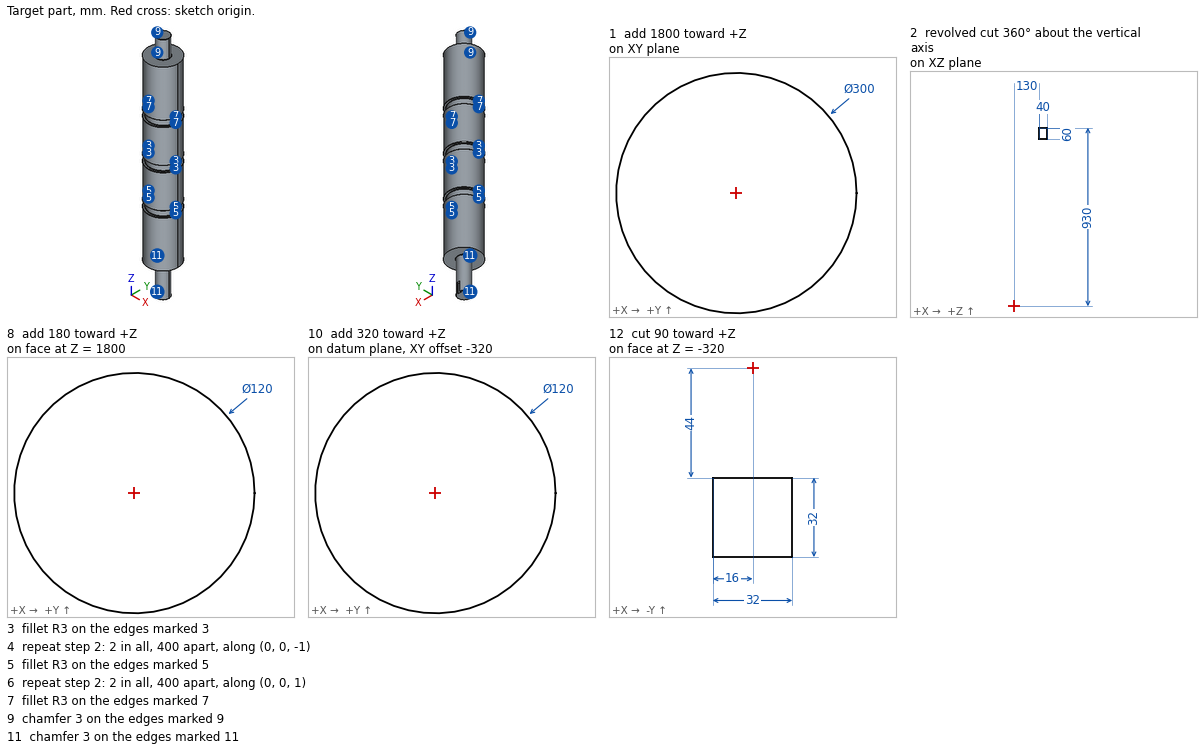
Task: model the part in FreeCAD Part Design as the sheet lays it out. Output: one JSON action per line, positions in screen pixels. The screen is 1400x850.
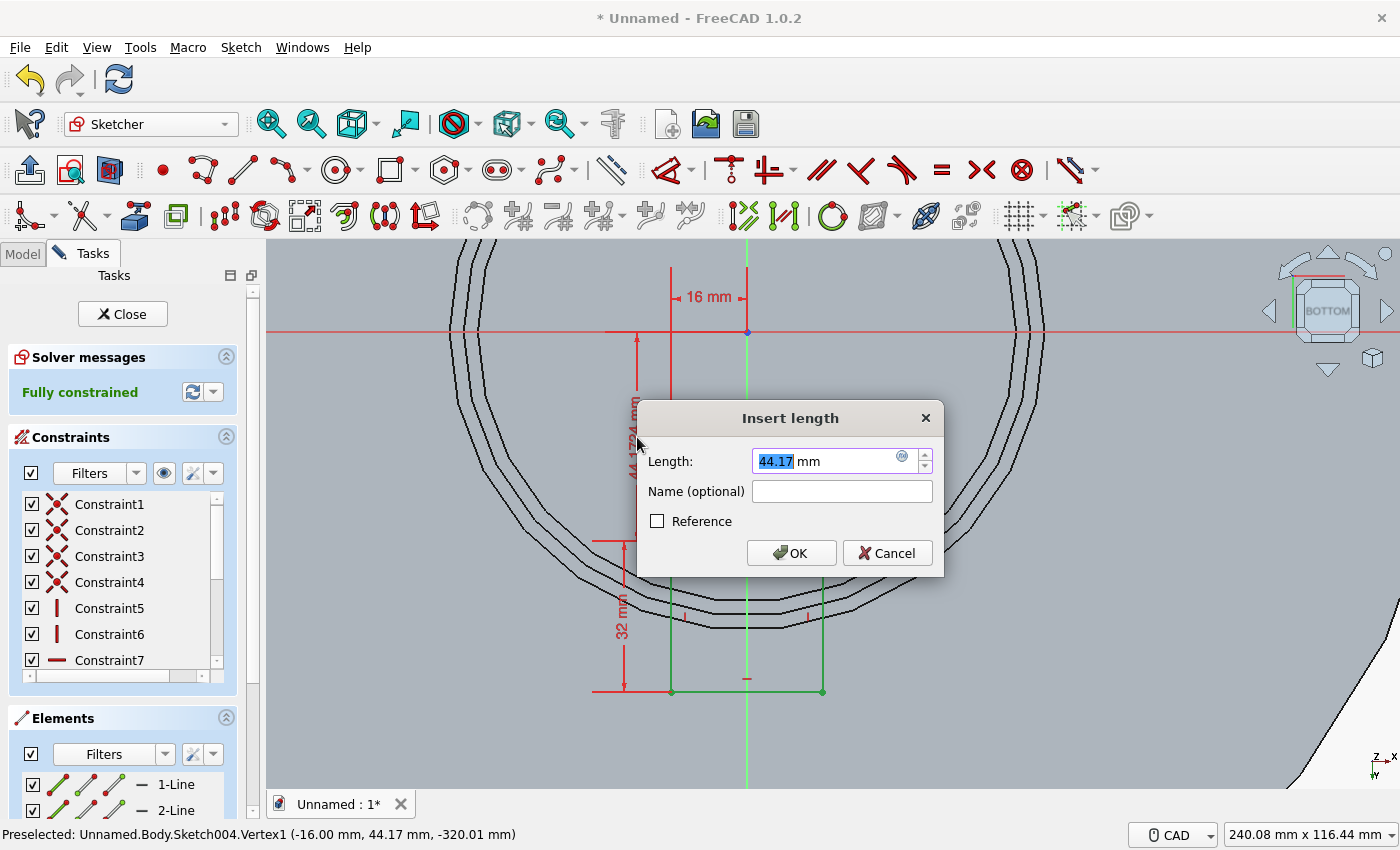
{"action": "type", "text": "44"}
{"action": "key", "text": "Return"}
{"action": "key", "text": "Escape"}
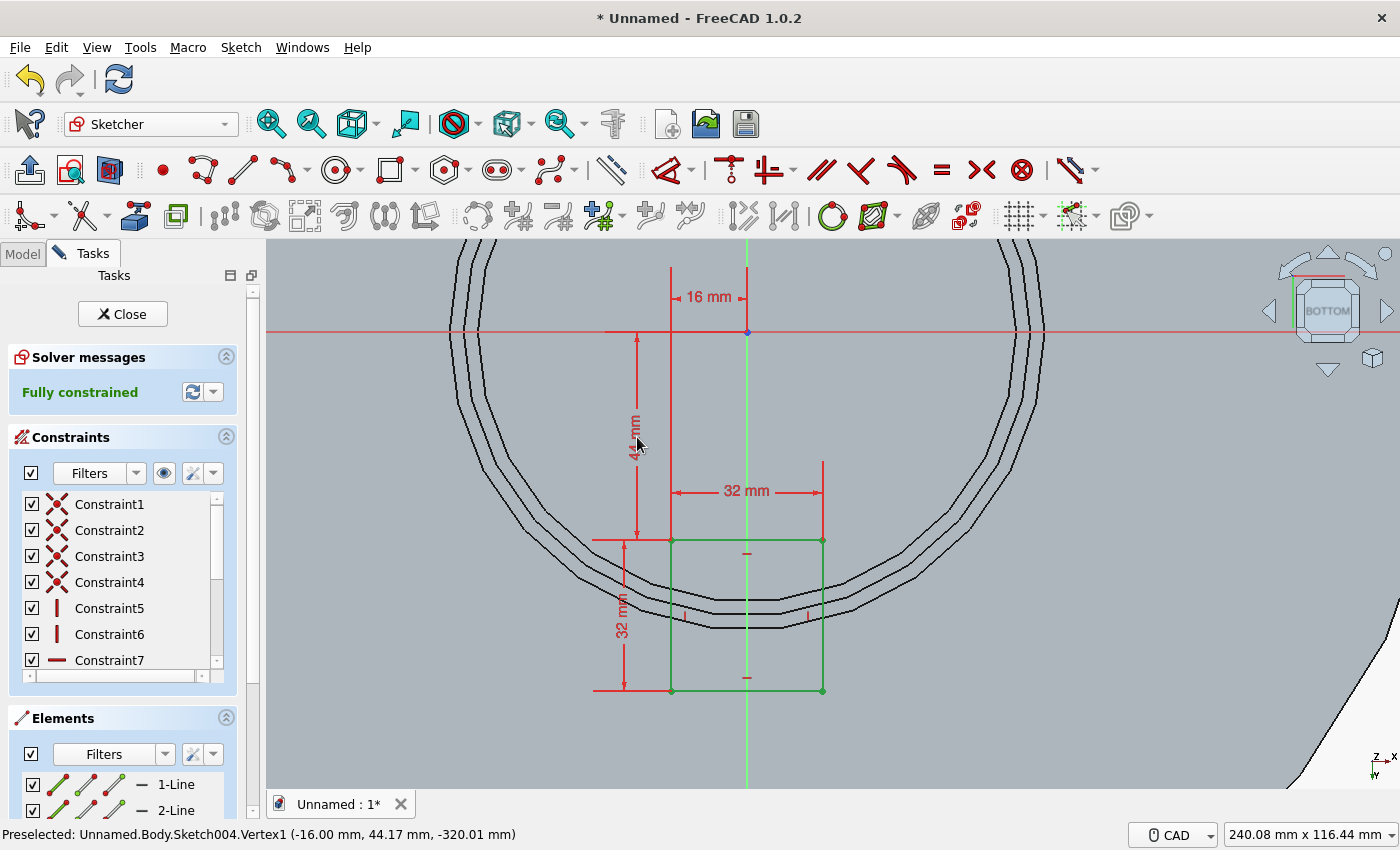
{"action": "left_click", "coordinate": [123, 314]}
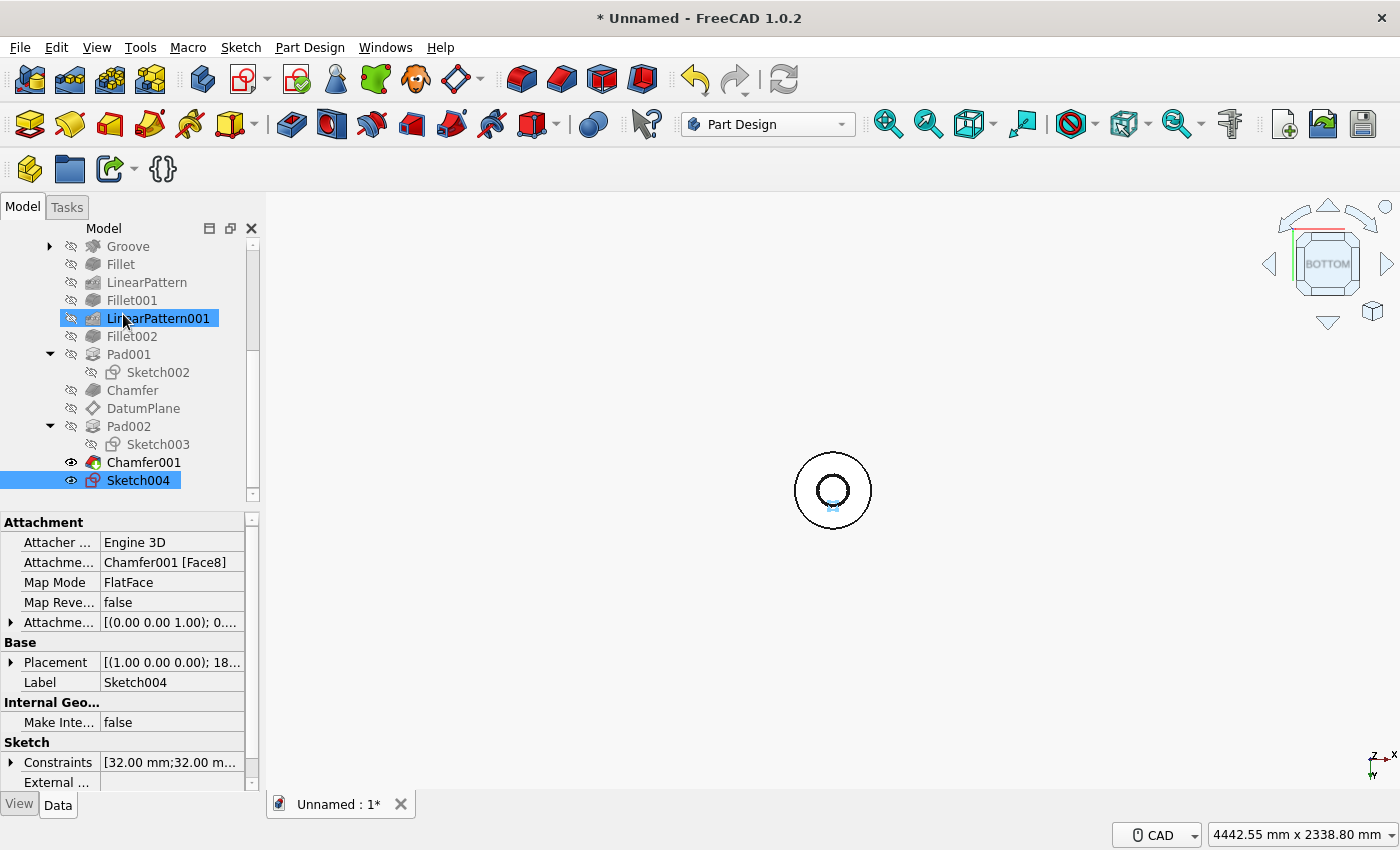
{"action": "left_click", "coordinate": [292, 124]}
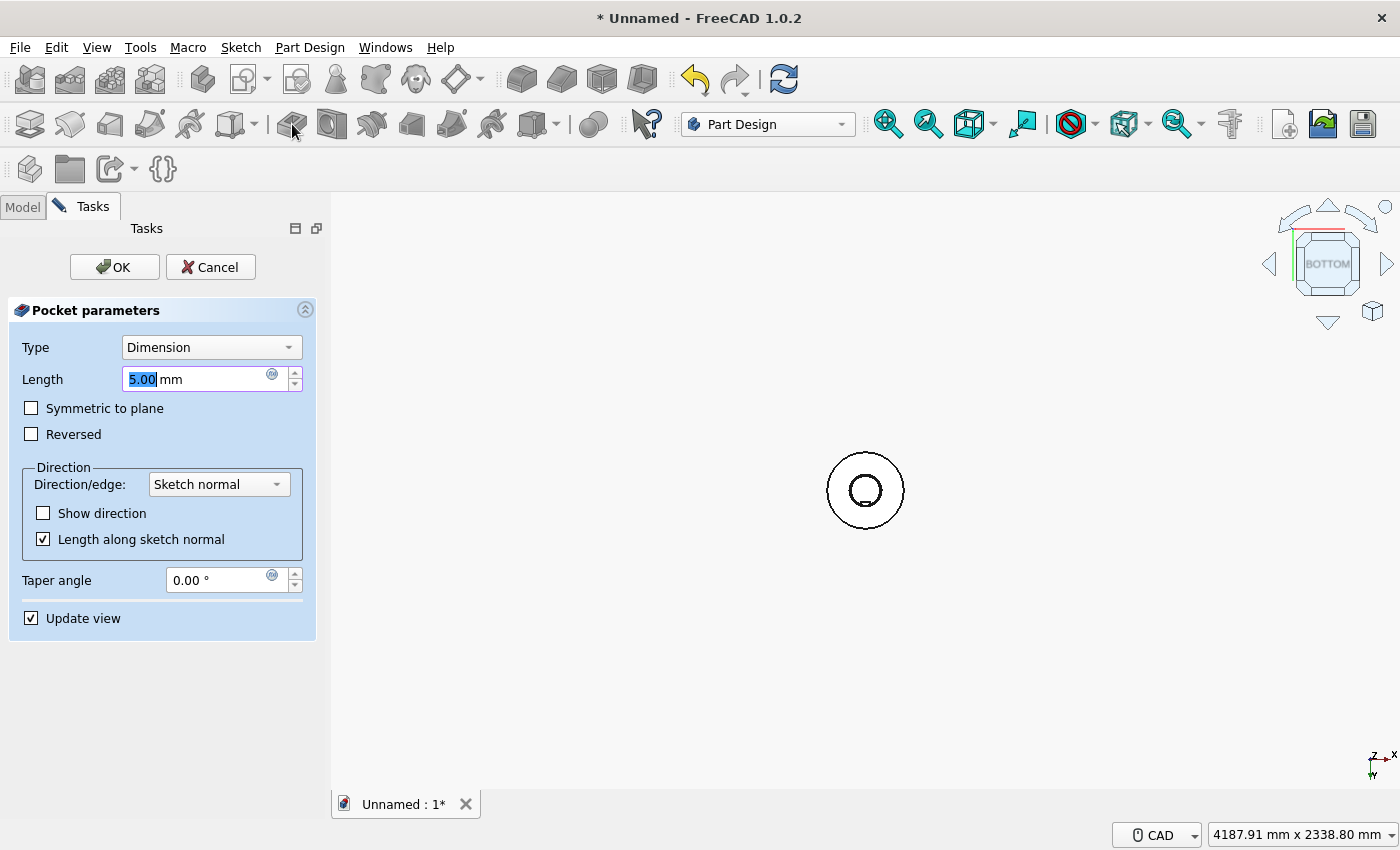
{"action": "type", "text": "90"}
{"action": "key", "text": "Tab"}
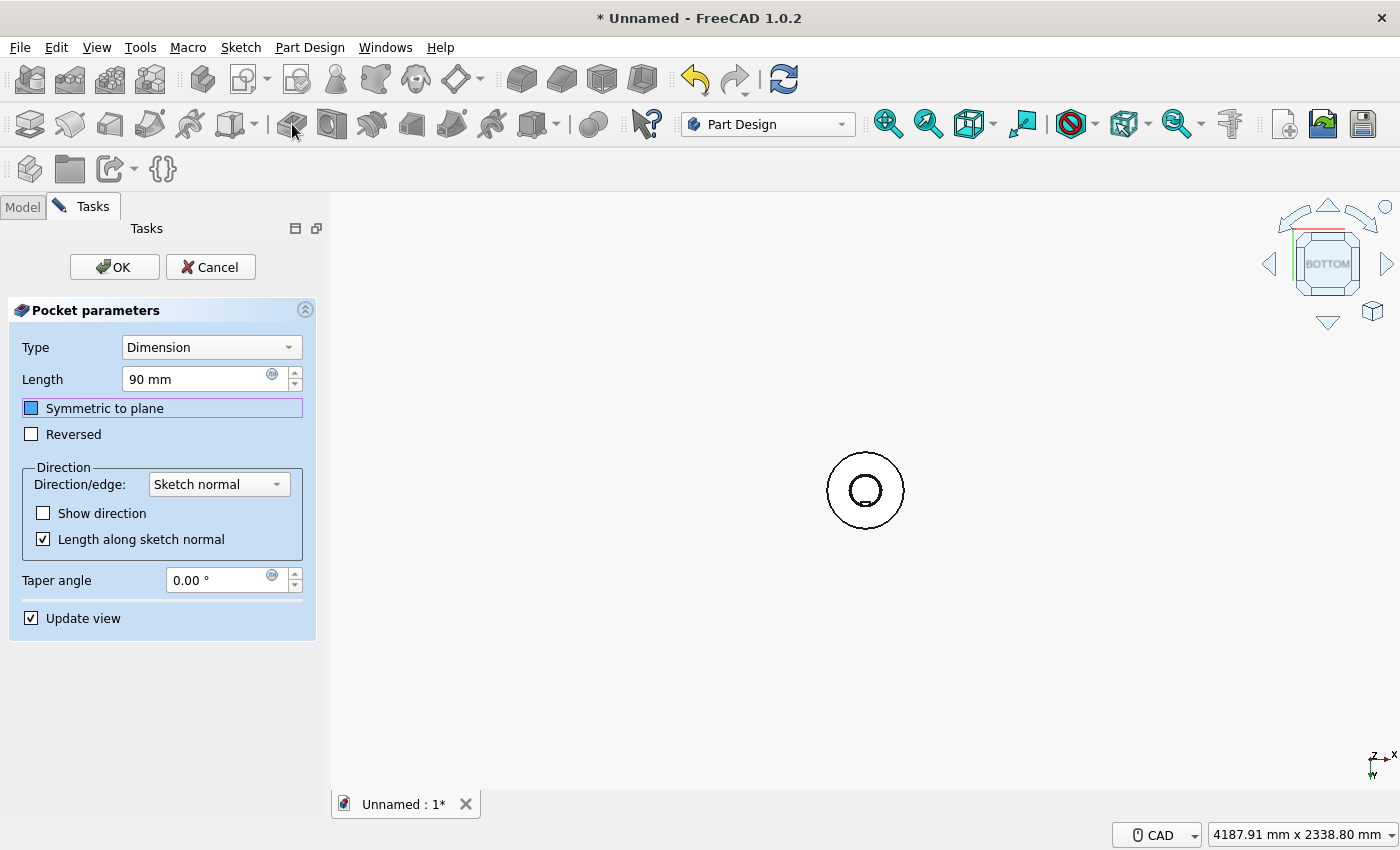
{"action": "left_click", "coordinate": [115, 267]}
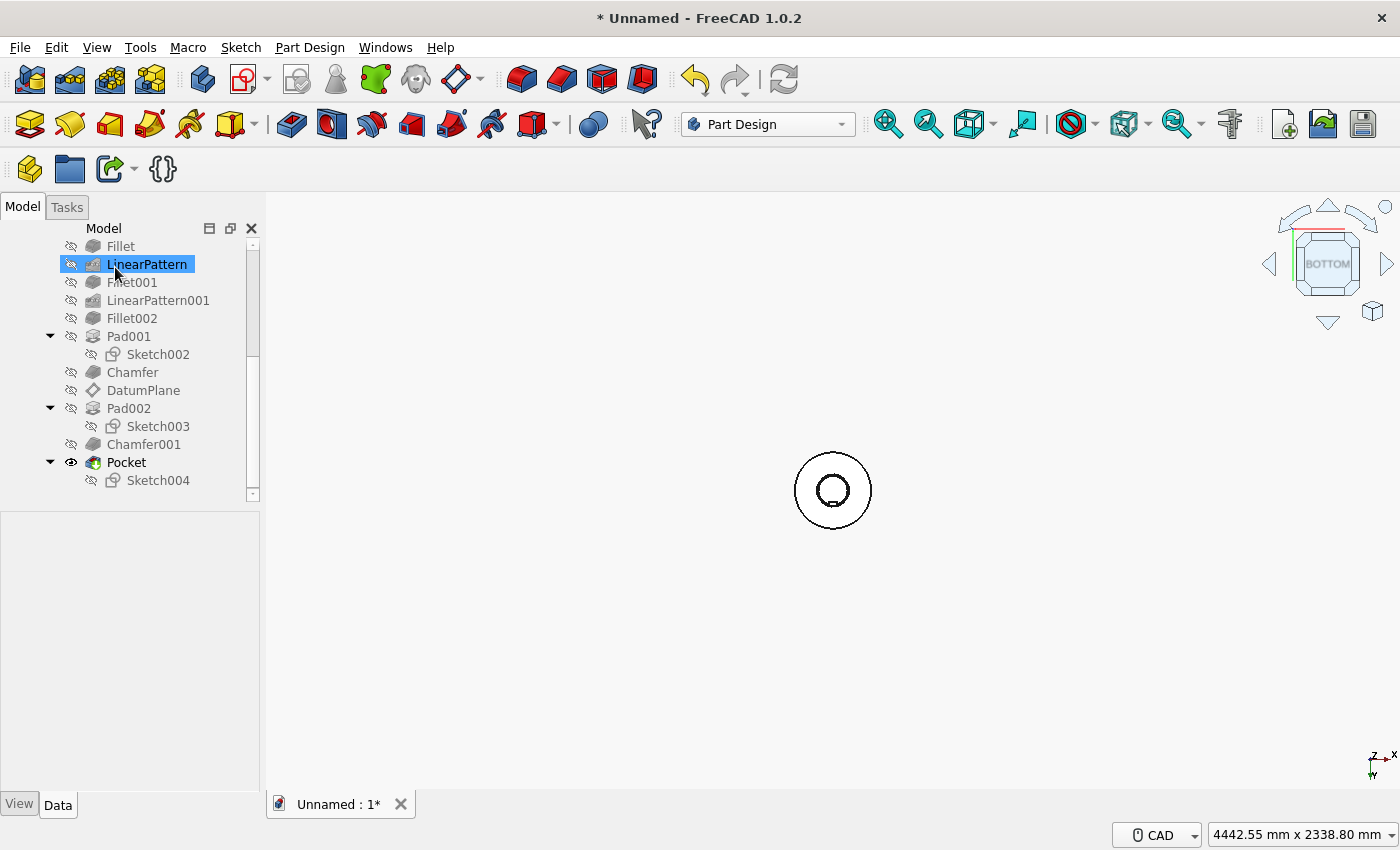
{"action": "key", "text": "0"}